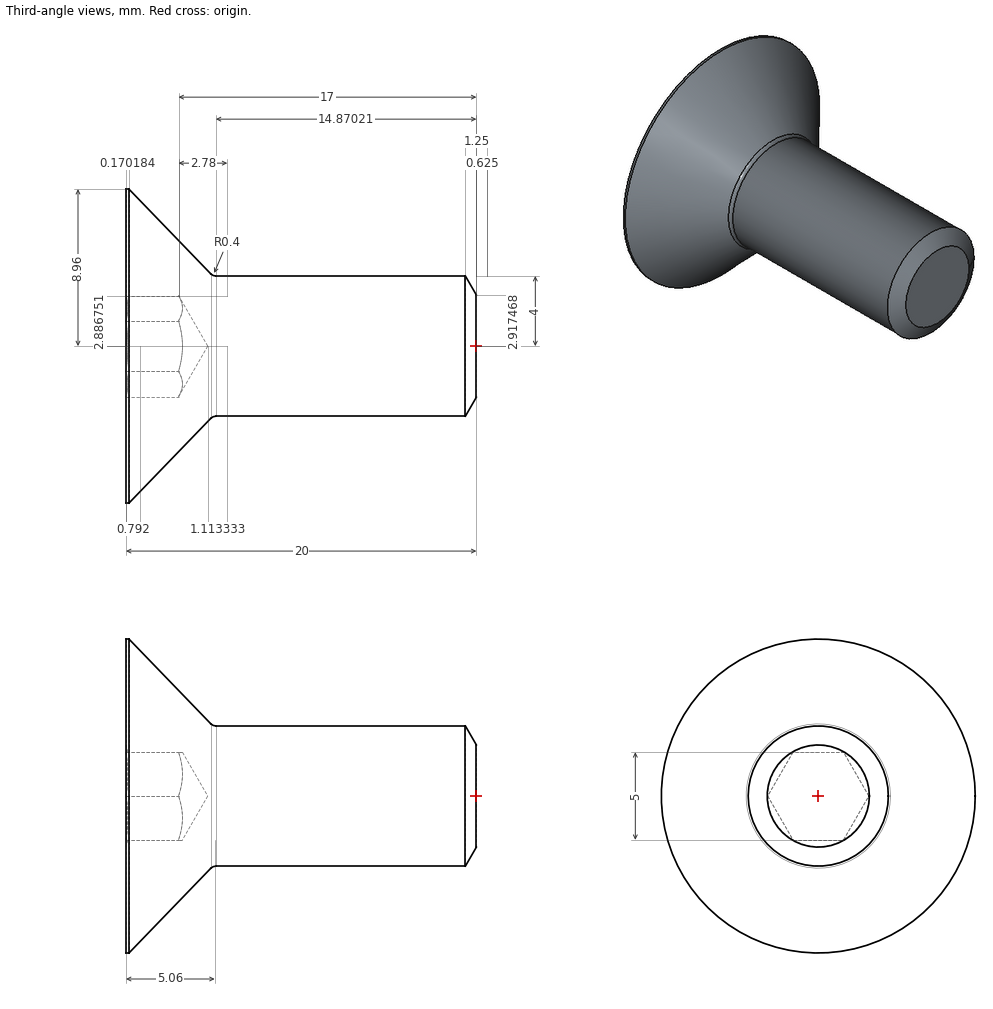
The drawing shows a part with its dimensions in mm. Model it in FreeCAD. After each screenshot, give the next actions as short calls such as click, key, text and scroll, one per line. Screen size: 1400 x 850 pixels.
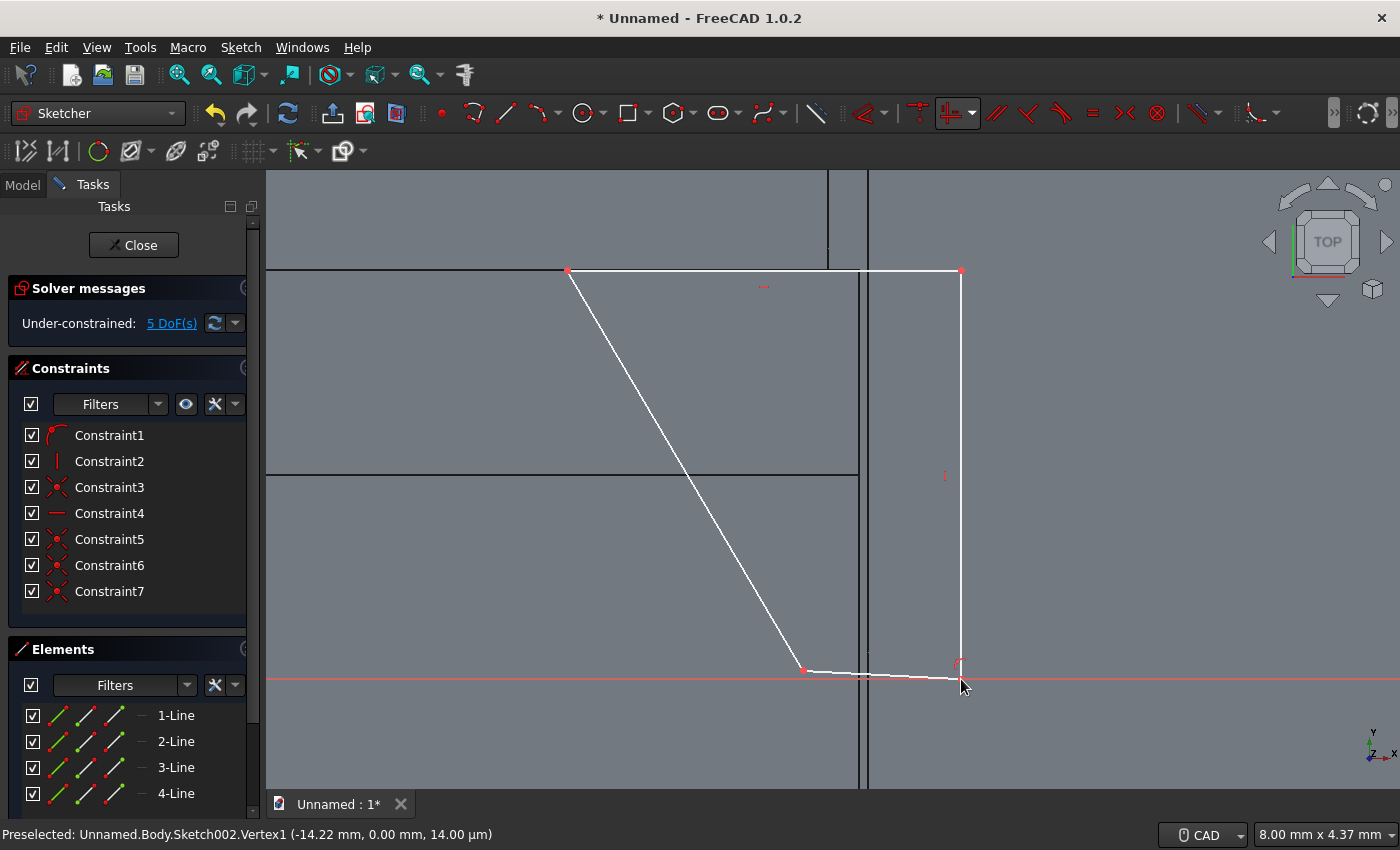
click(914, 677)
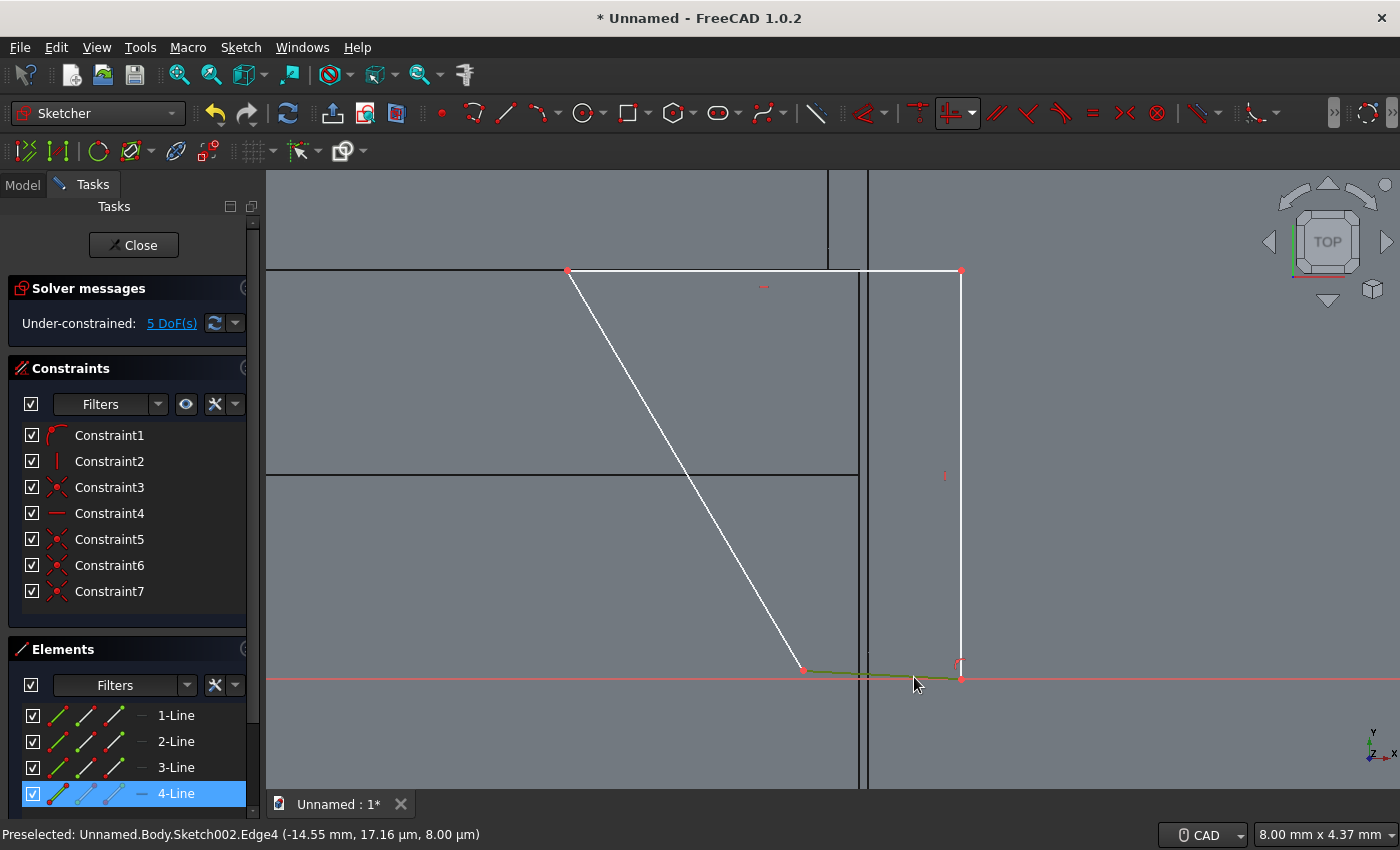
click(974, 114)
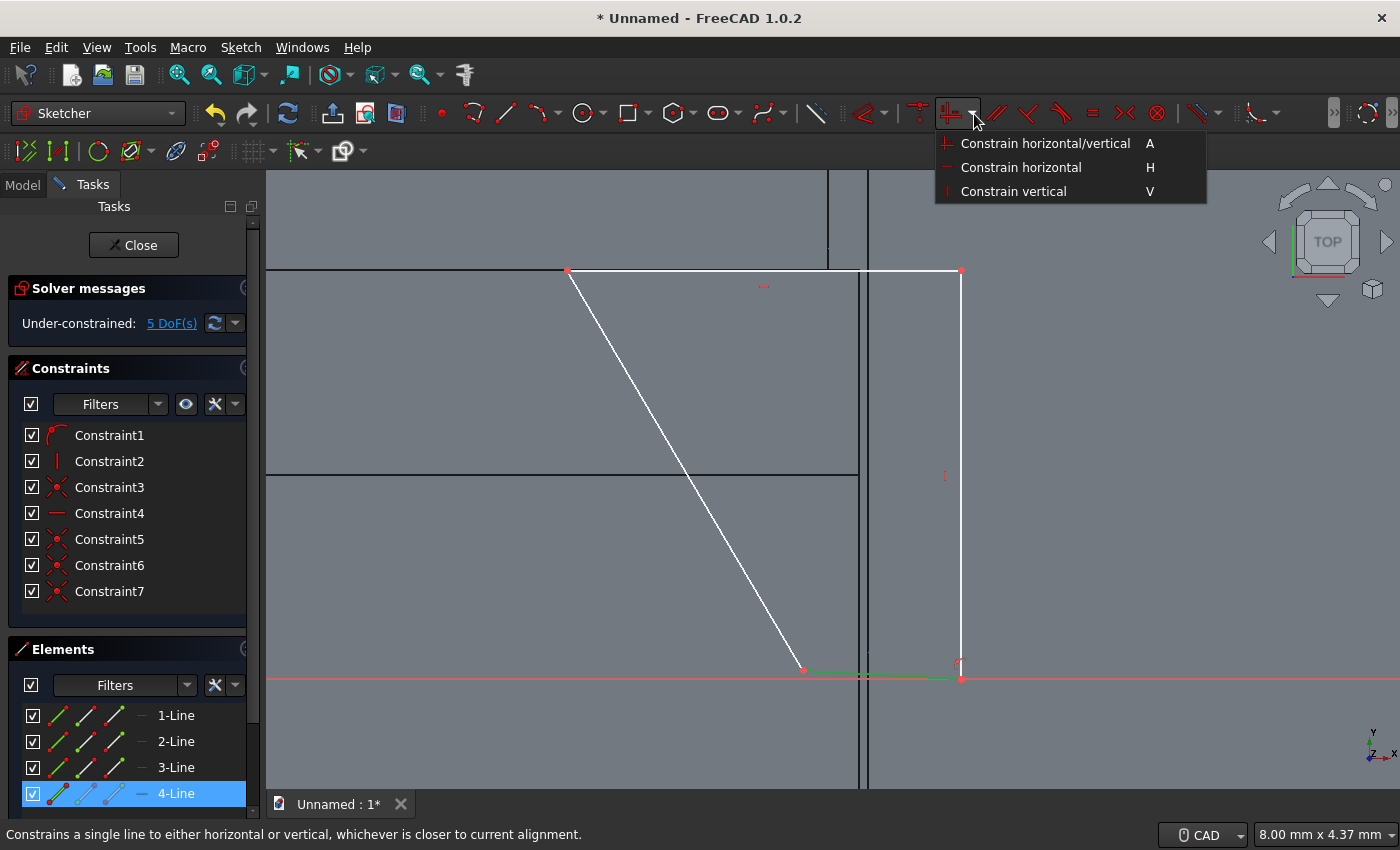
click(1071, 167)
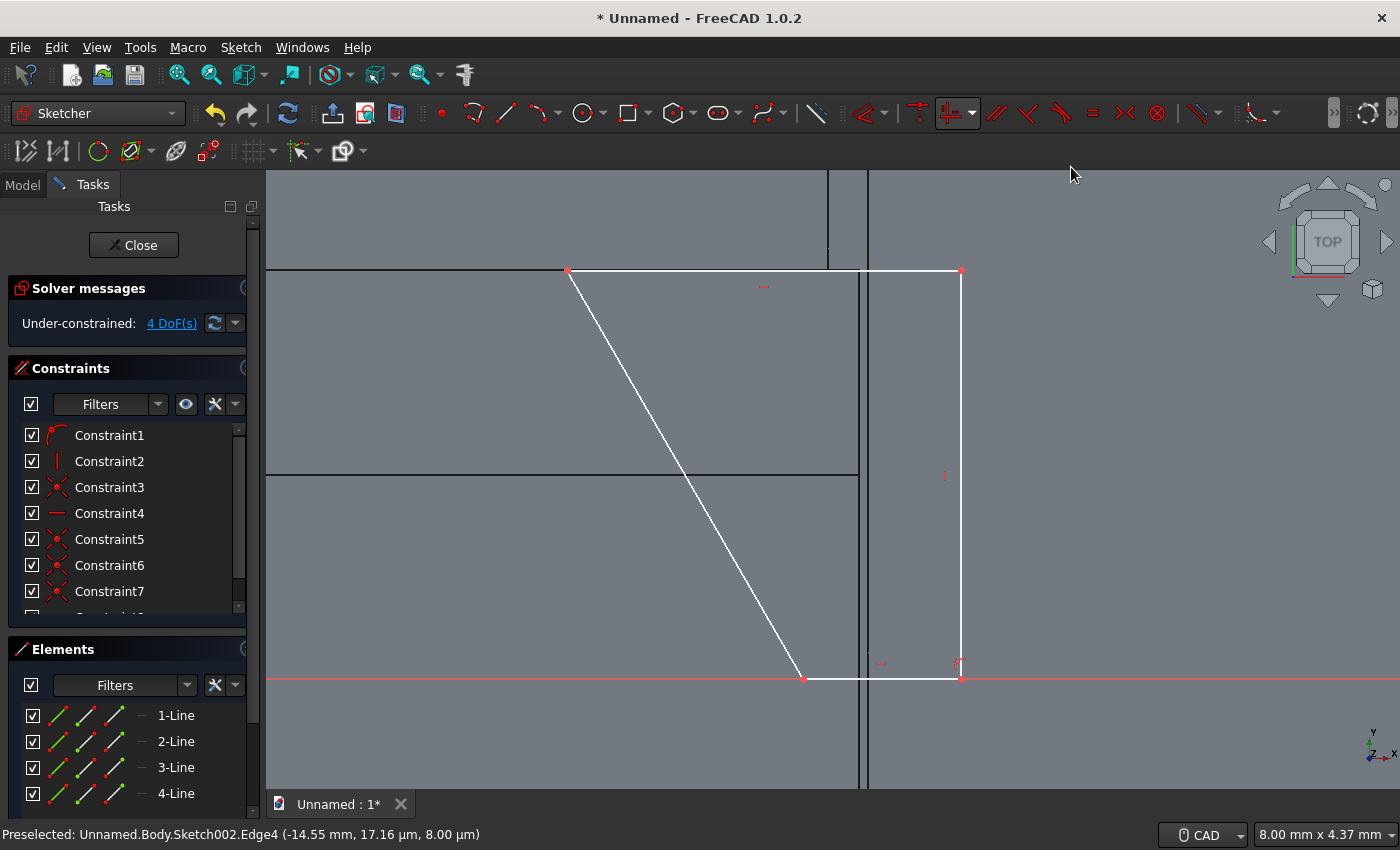
click(864, 114)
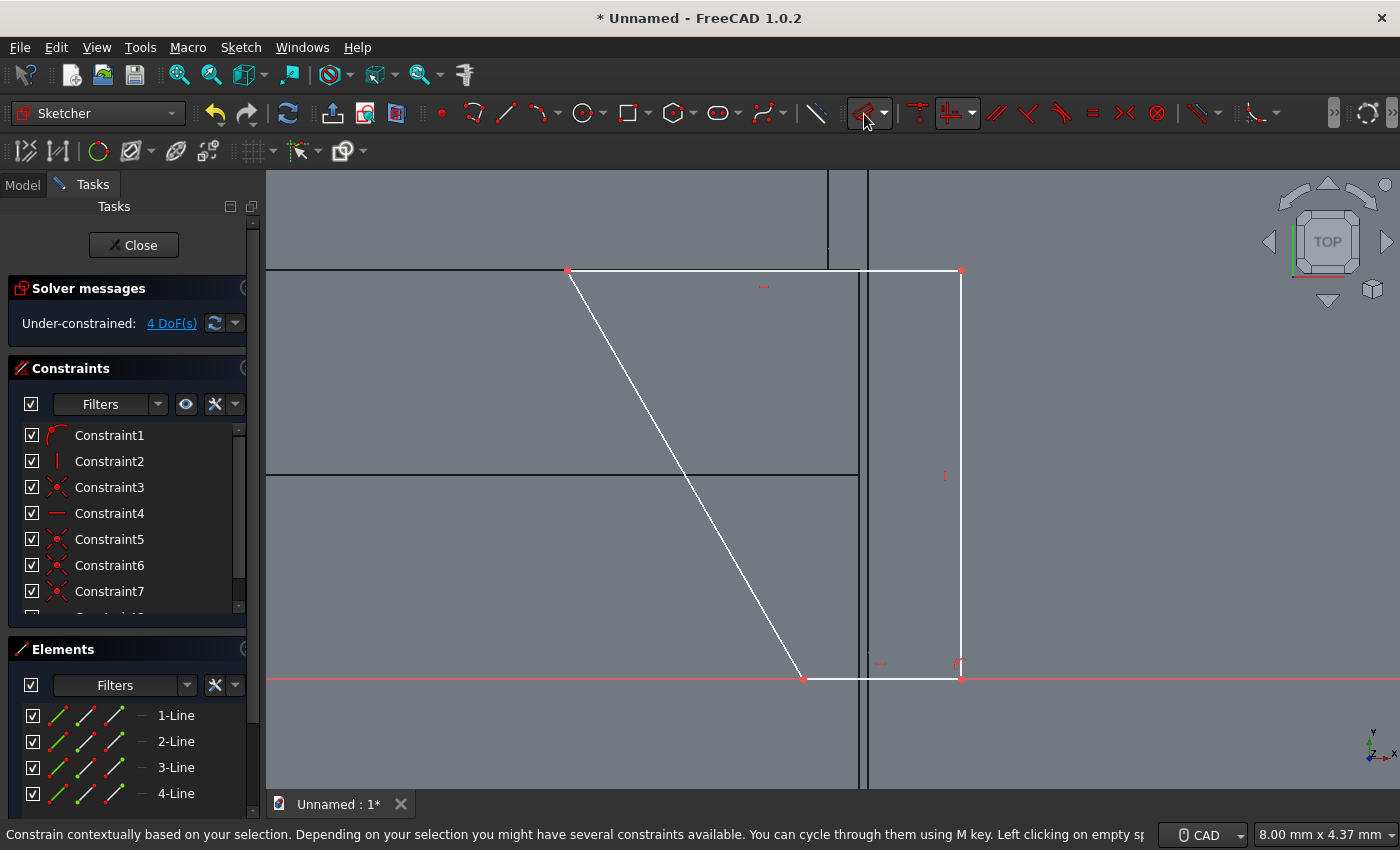
click(567, 271)
click(901, 713)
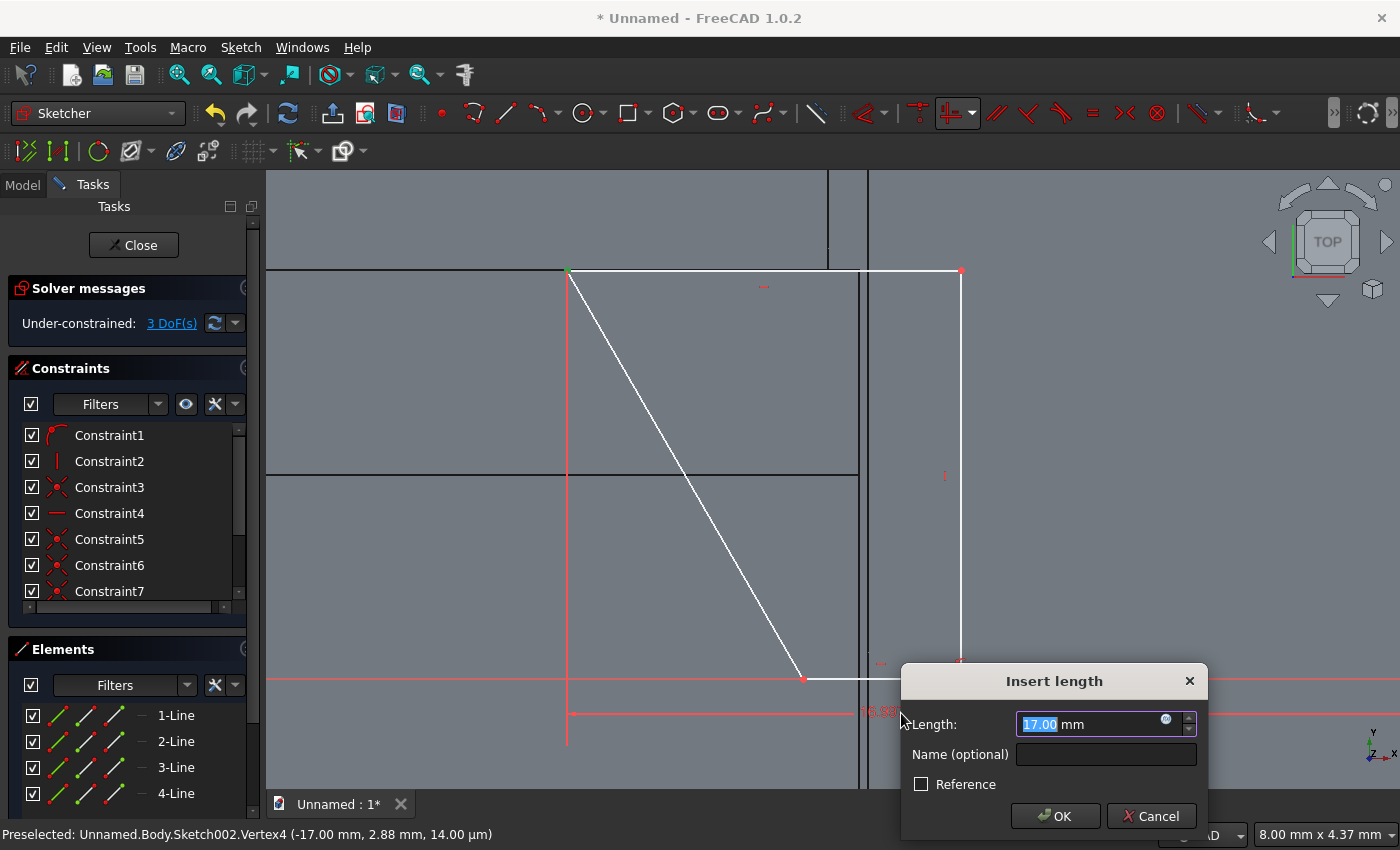
text(17)
key(Return)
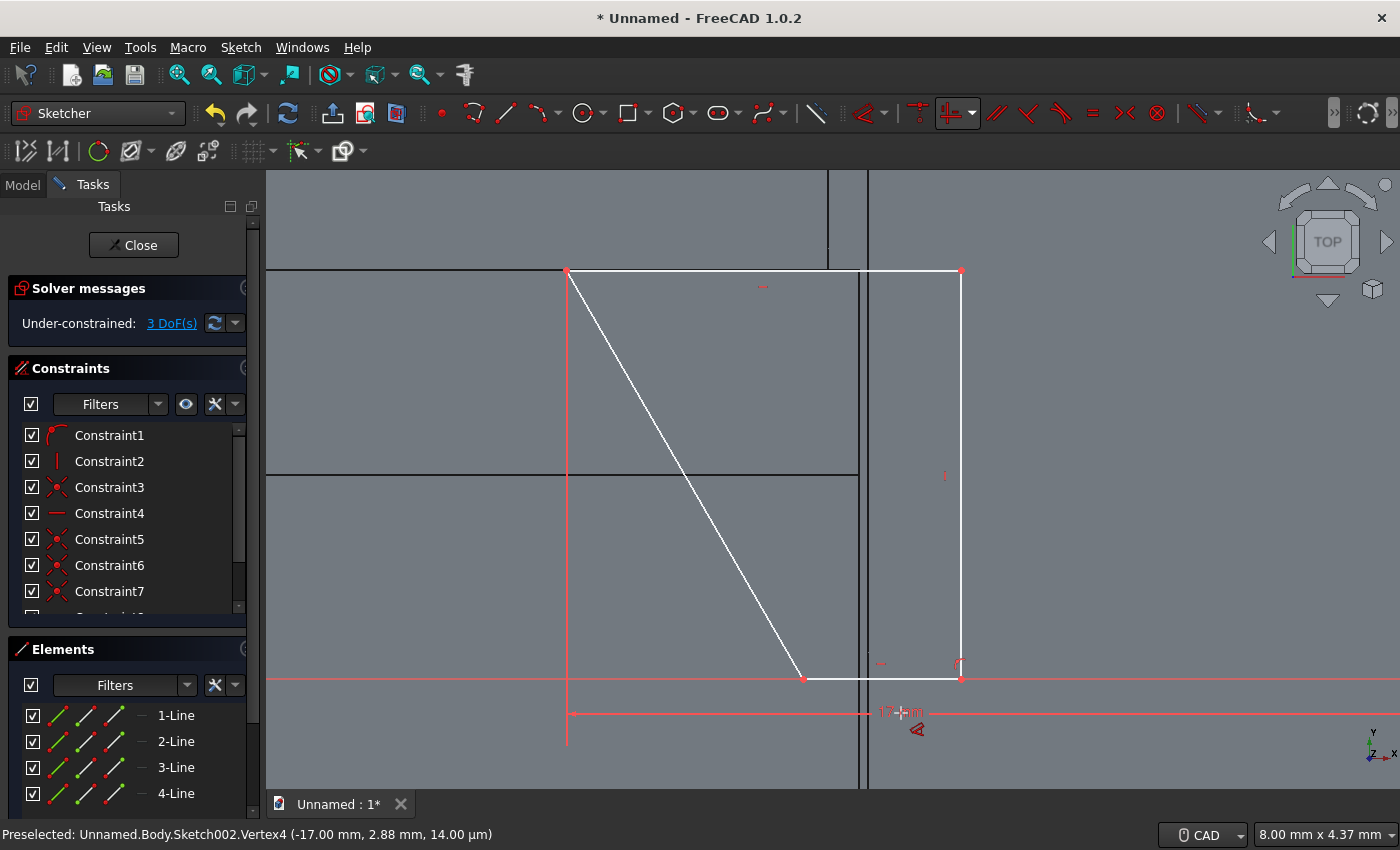
click(843, 271)
click(764, 237)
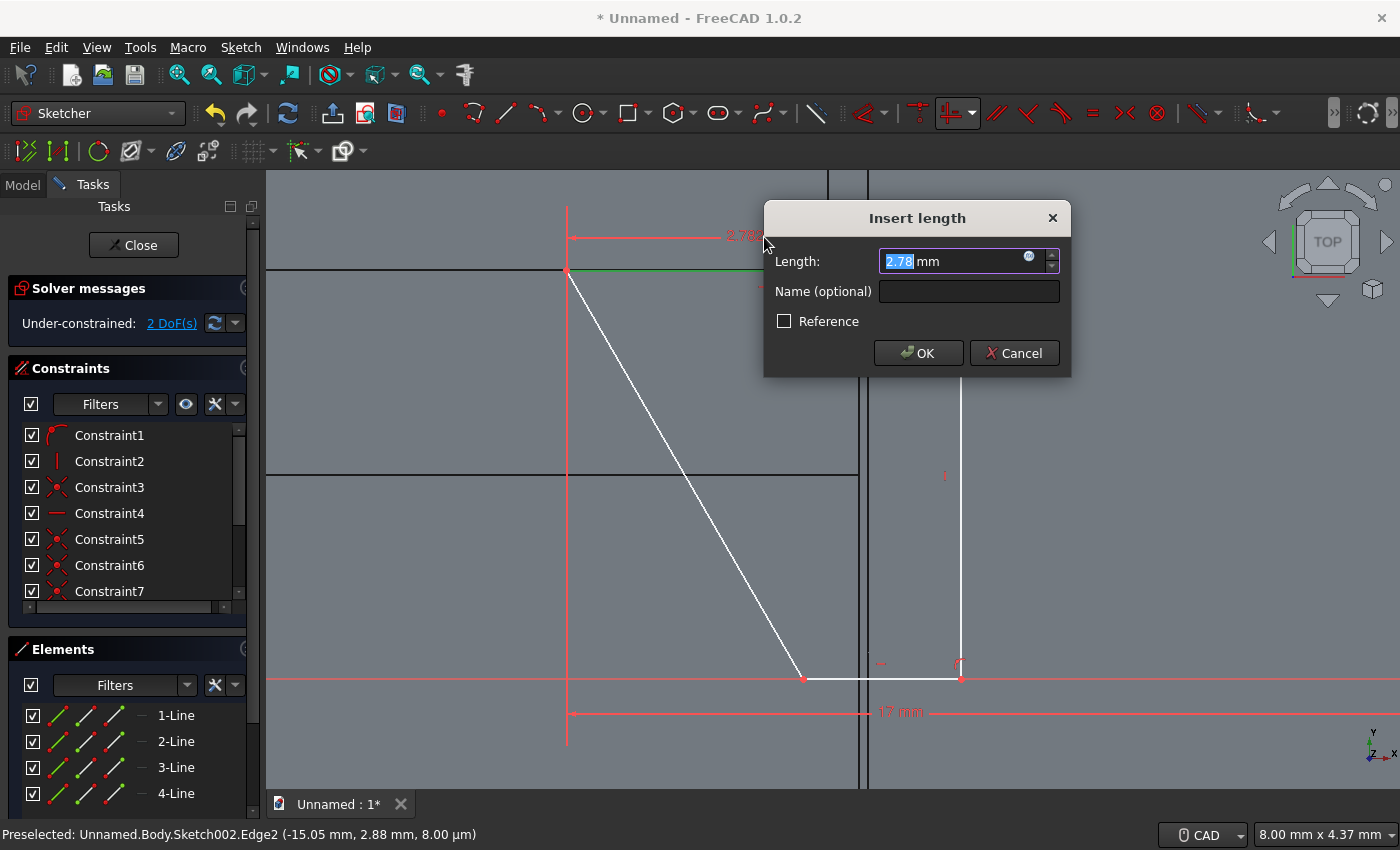
text(2.78)
key(Return)